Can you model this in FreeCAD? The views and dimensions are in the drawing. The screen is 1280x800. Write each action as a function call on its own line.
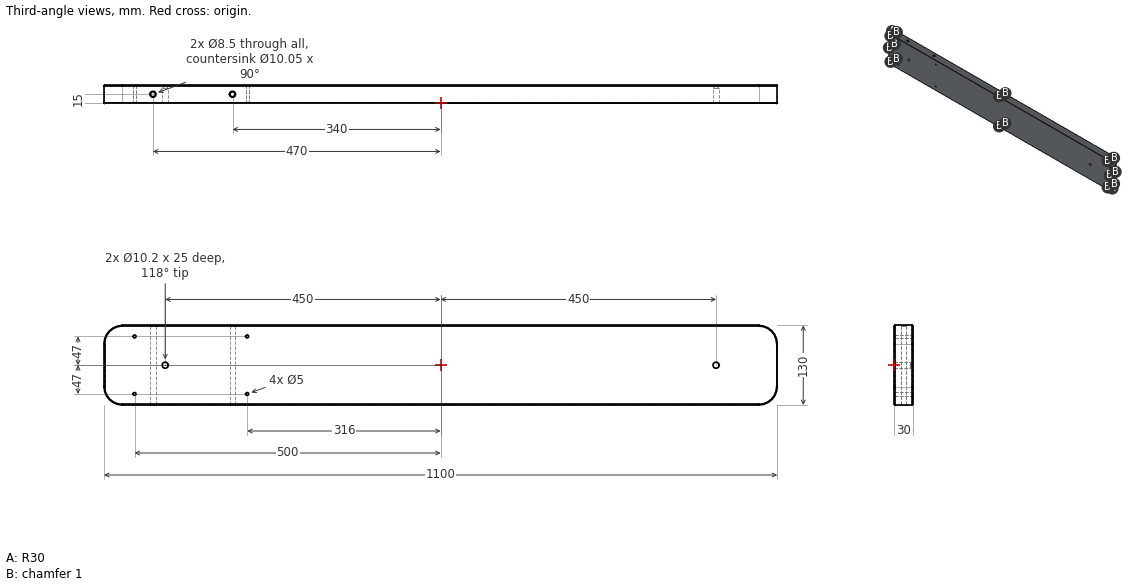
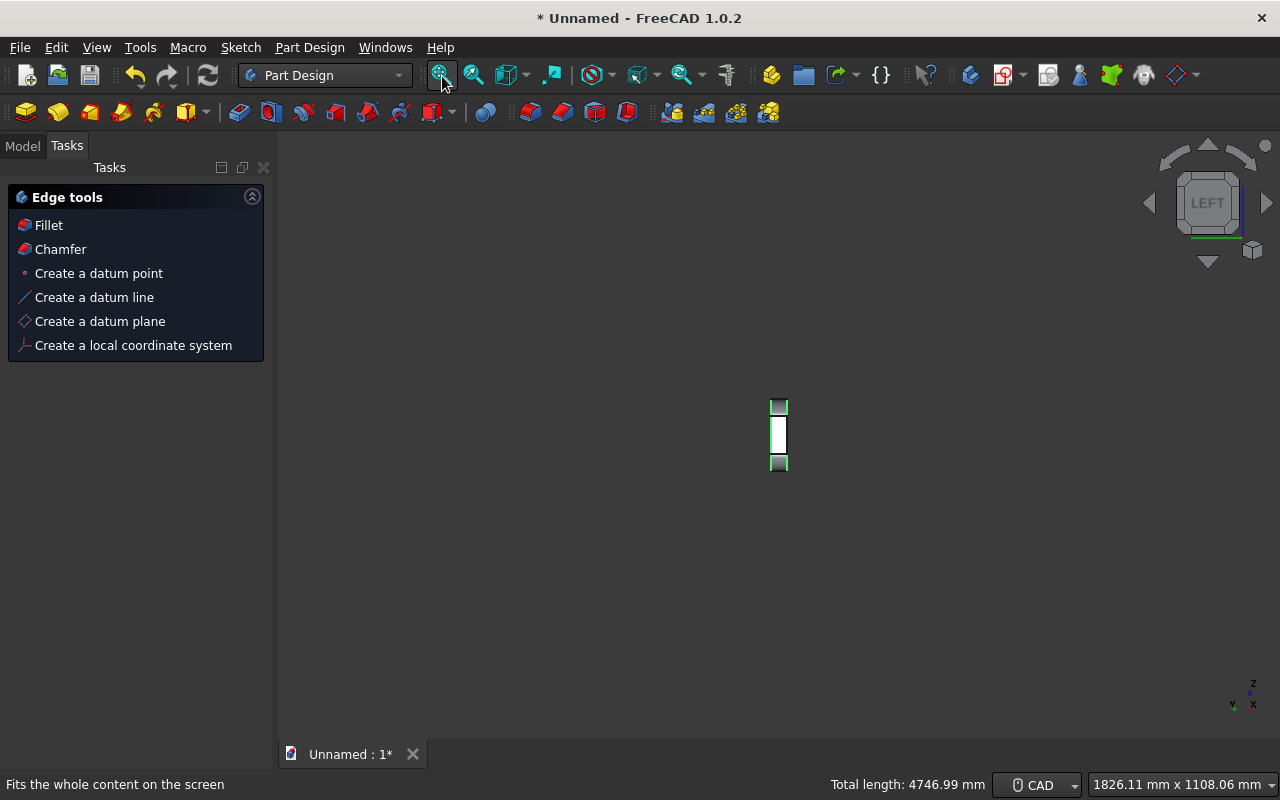
click(787, 434, ctrl)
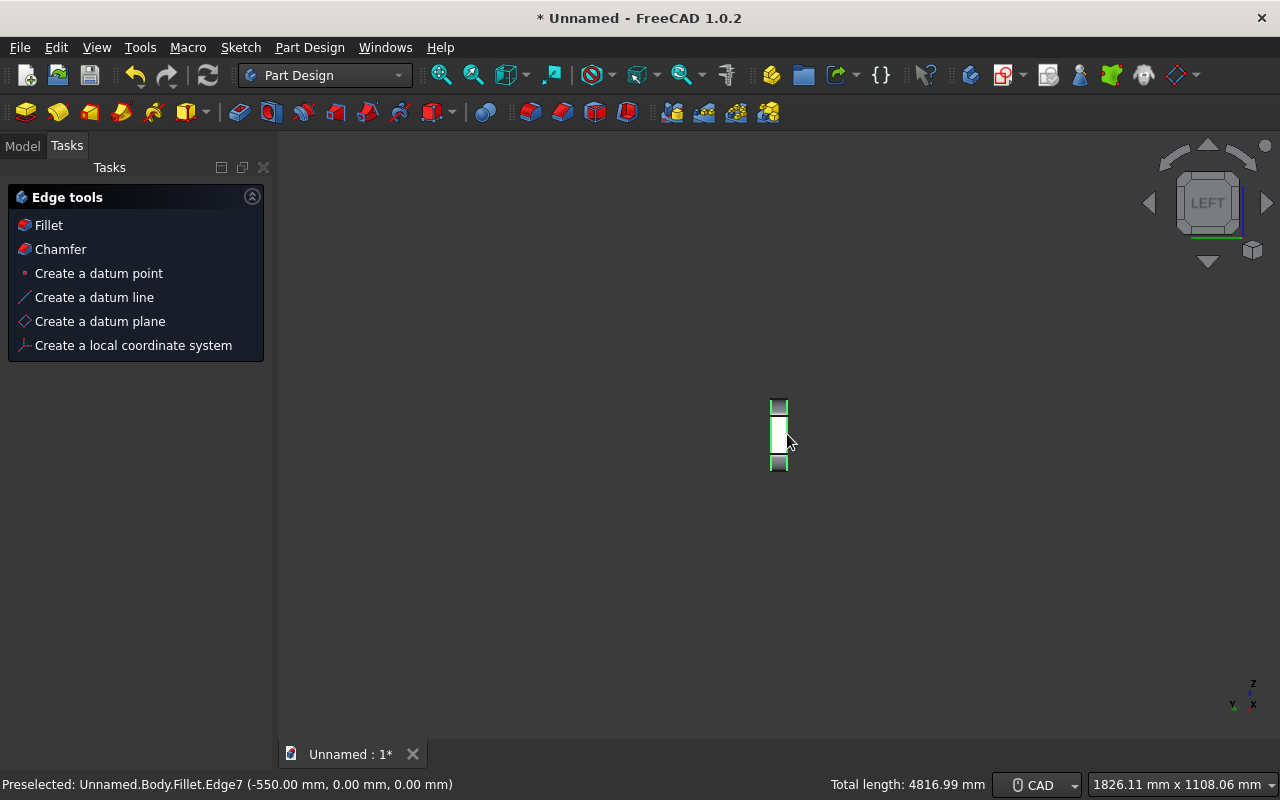
click(564, 112)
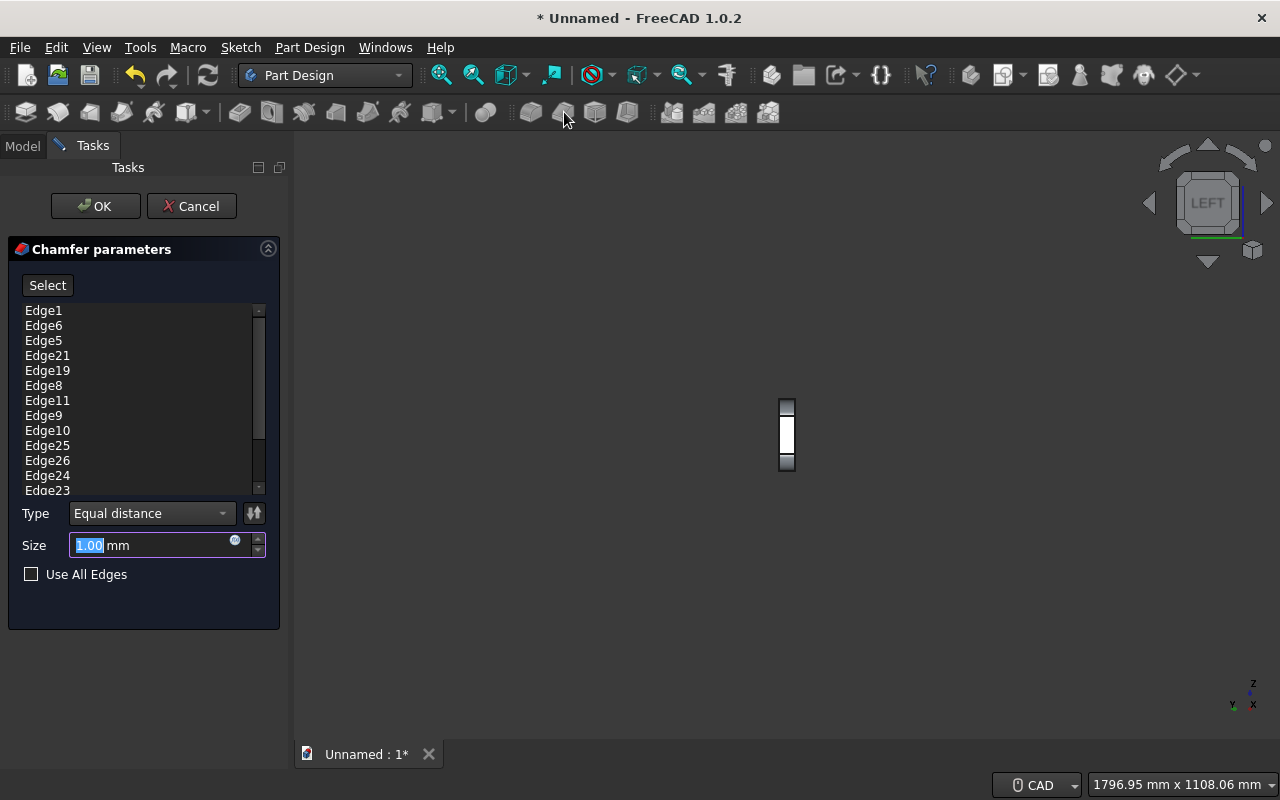
text(1)
key(Tab)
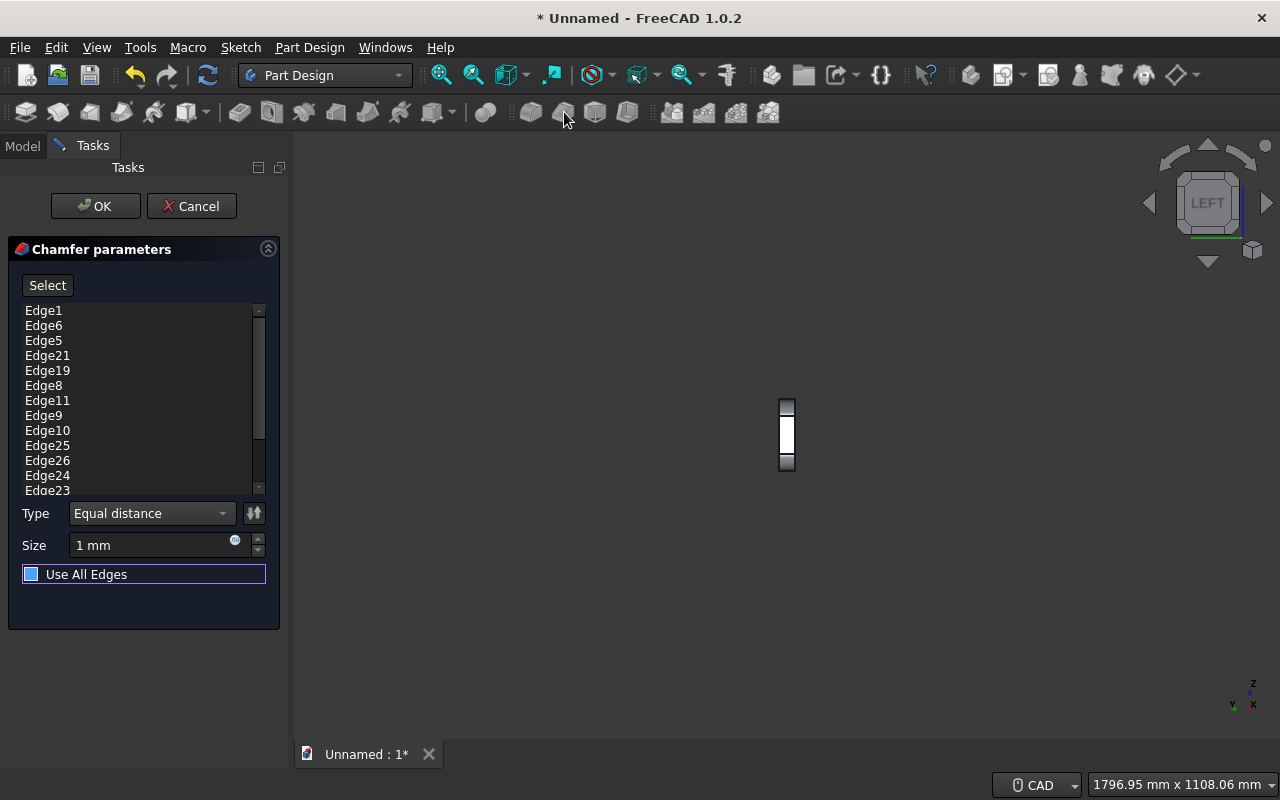
click(96, 206)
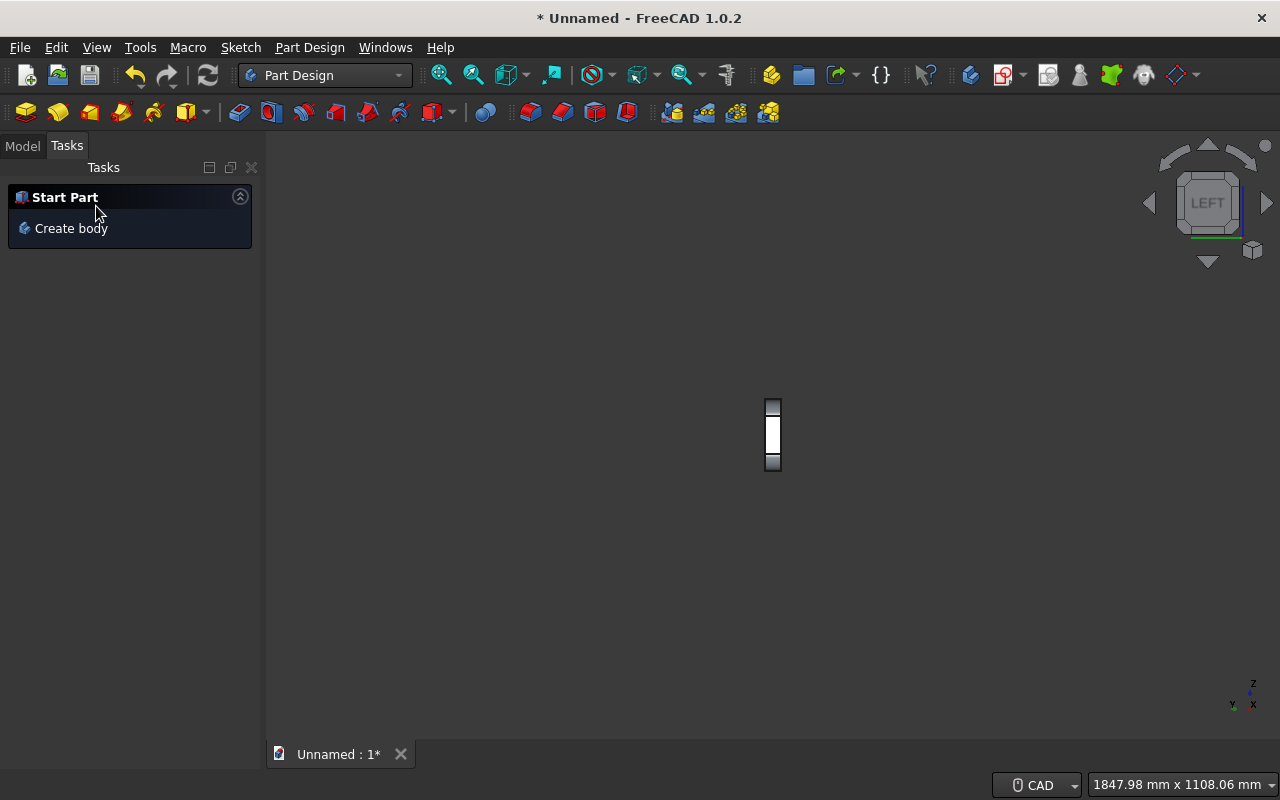
click(442, 76)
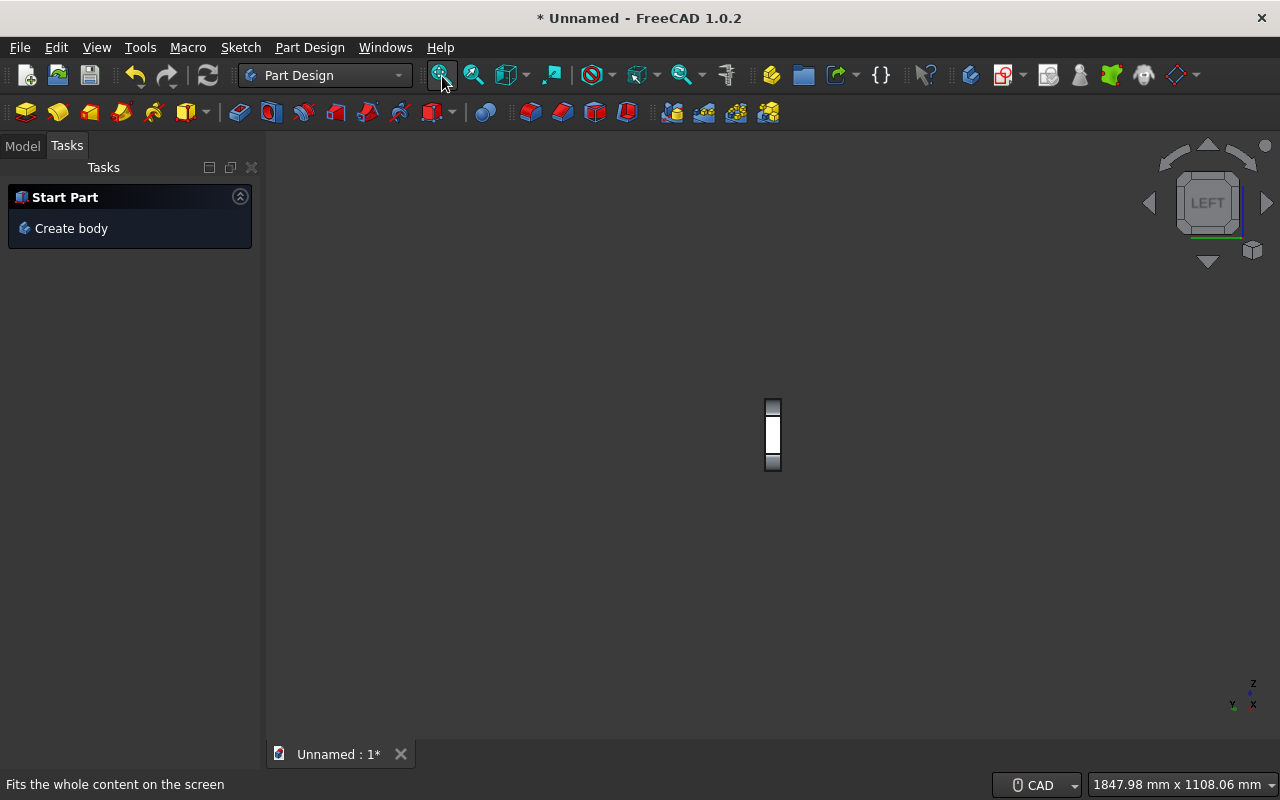
key(0)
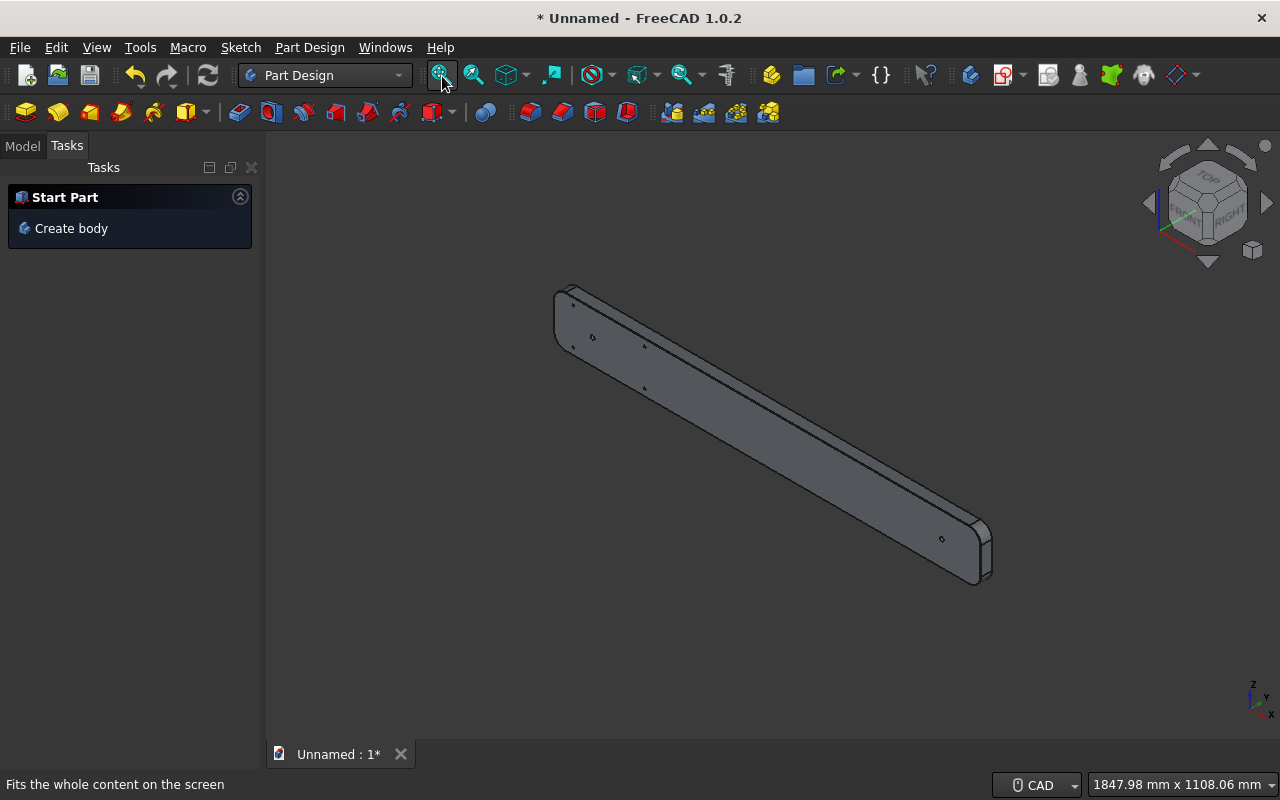
key(2)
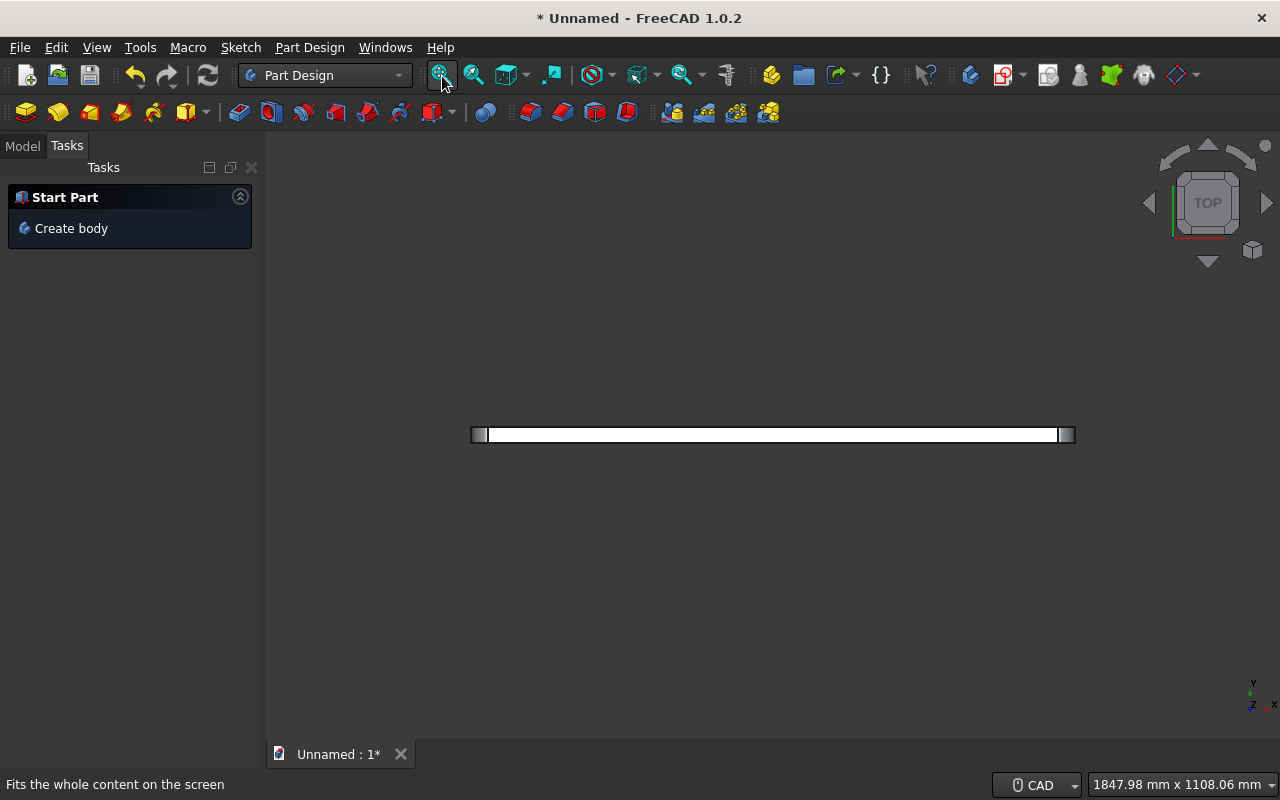
click(1018, 436)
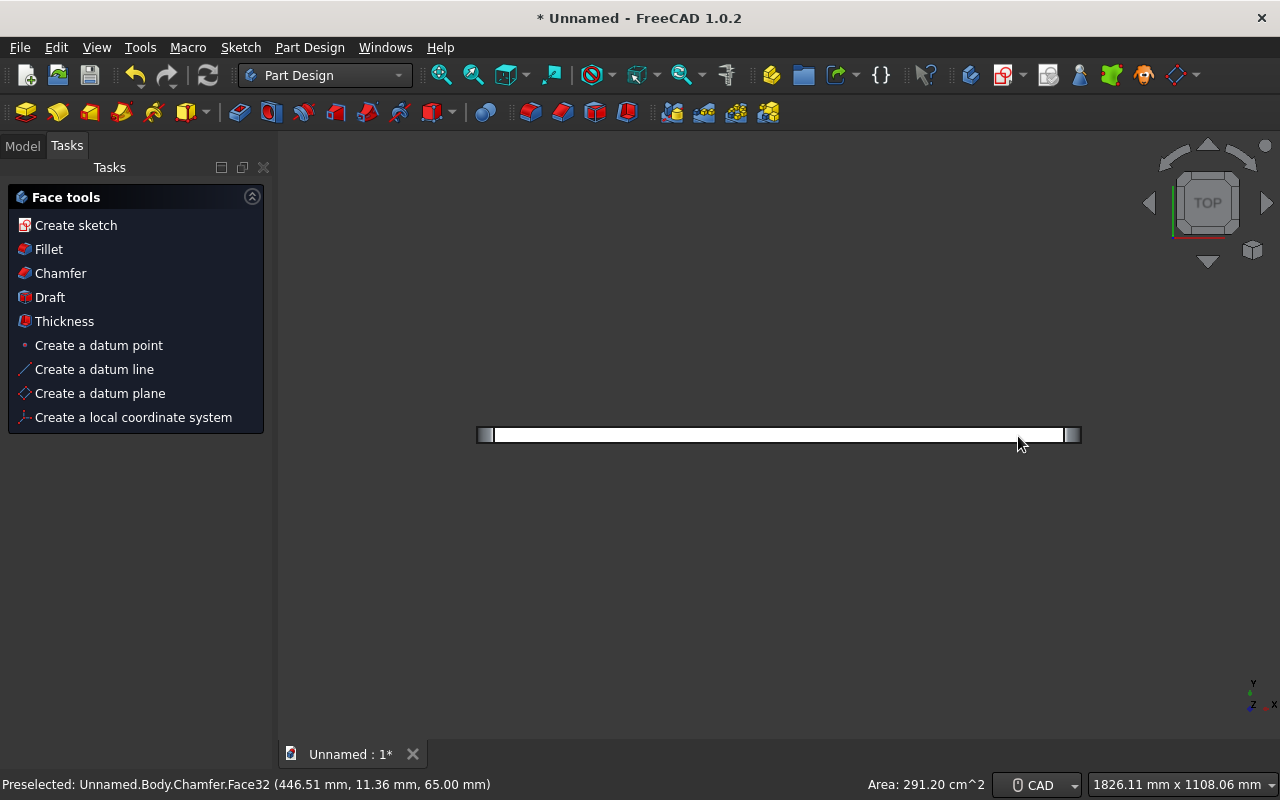
click(1004, 76)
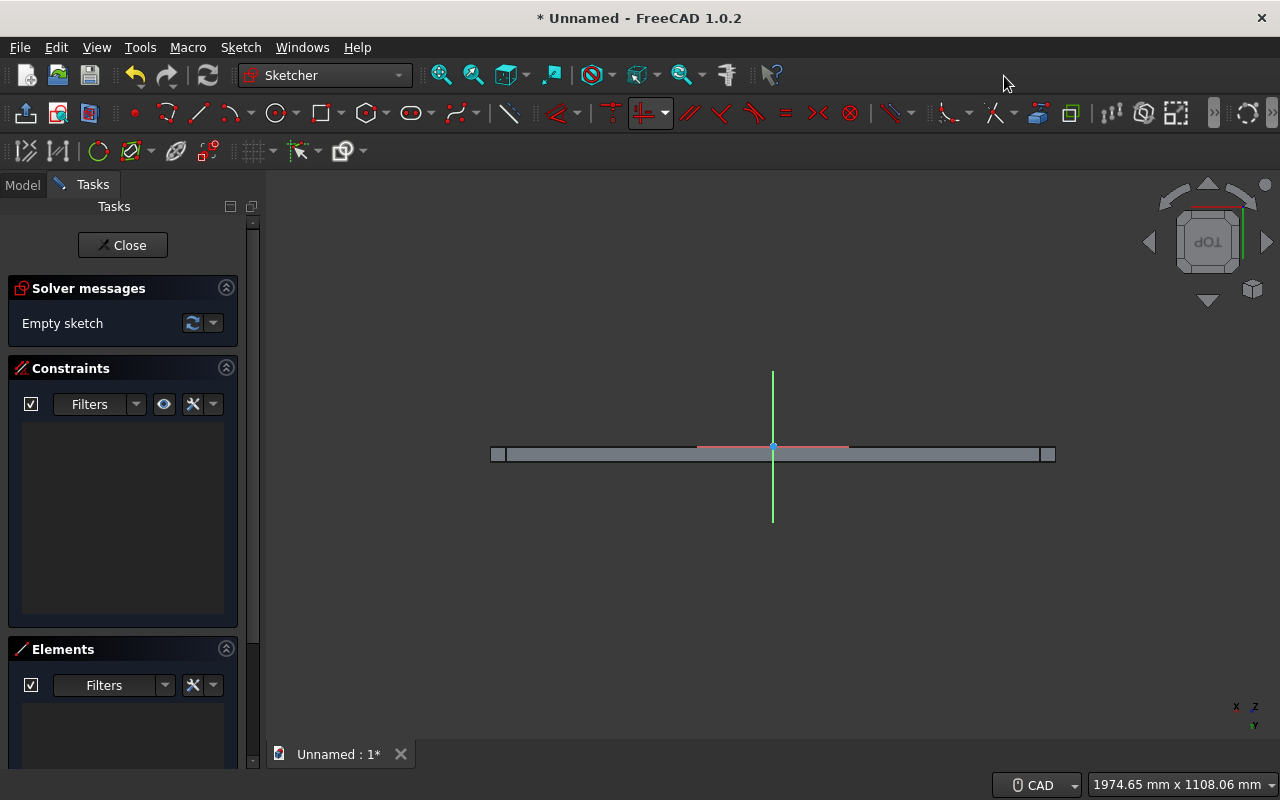
scroll(1024, 454, up, 10)